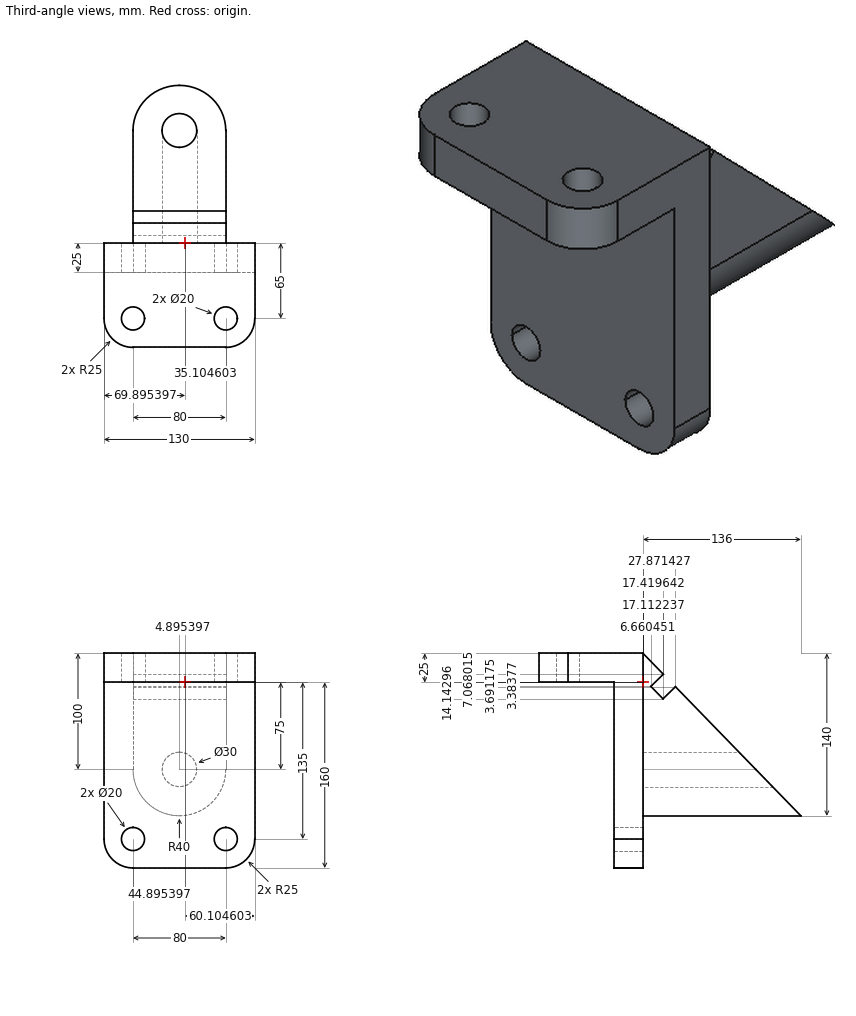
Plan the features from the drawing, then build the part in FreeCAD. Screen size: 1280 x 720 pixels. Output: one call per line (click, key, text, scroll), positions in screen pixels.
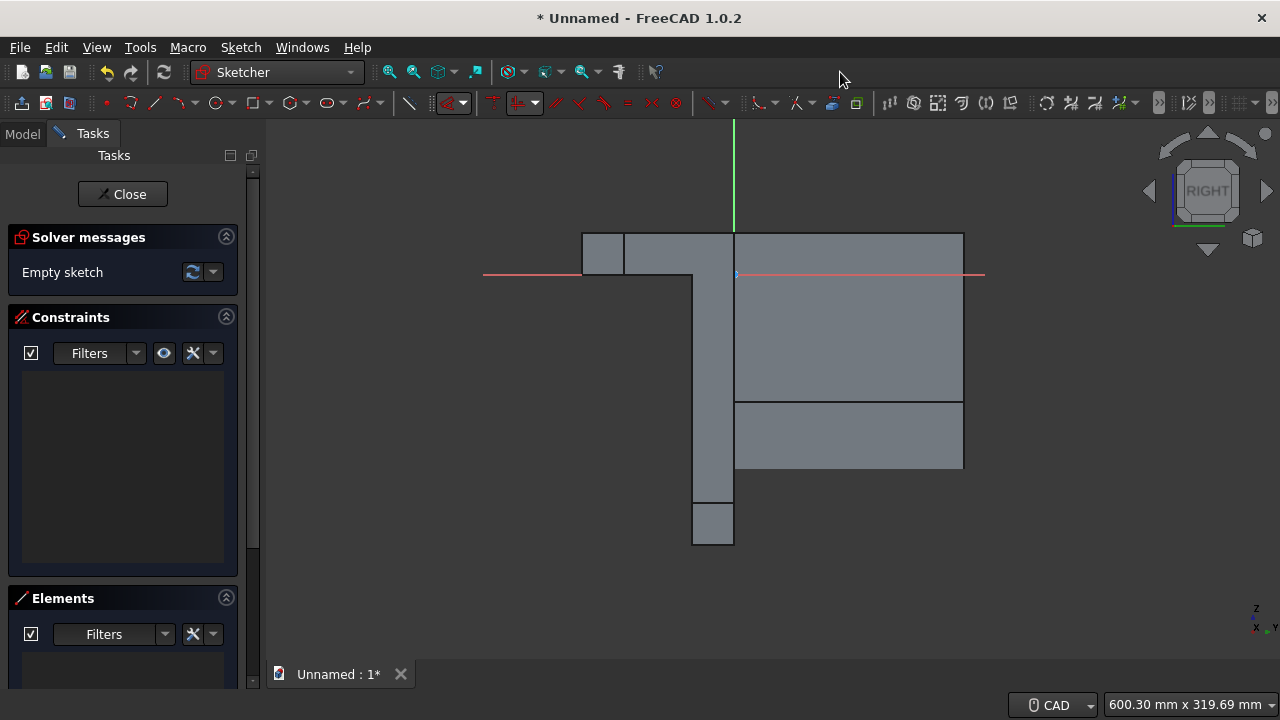
click(70, 104)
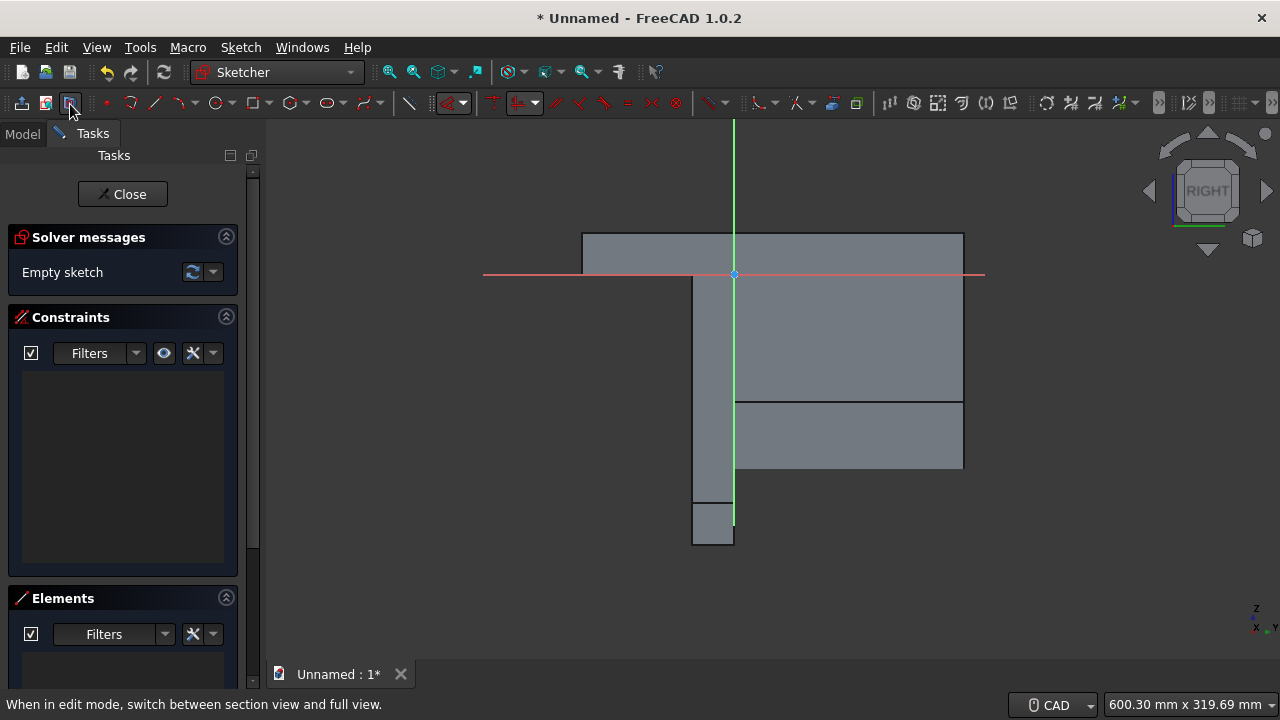
scroll(1115, 274, up, 2)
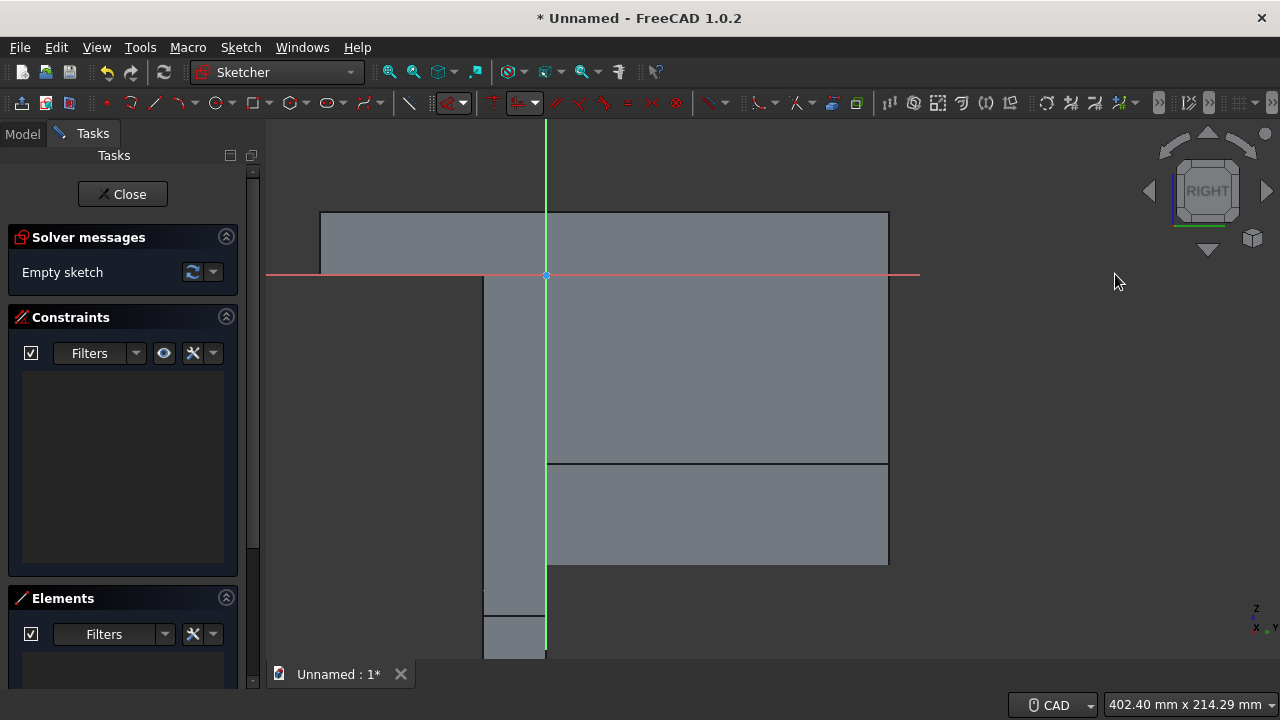
click(132, 104)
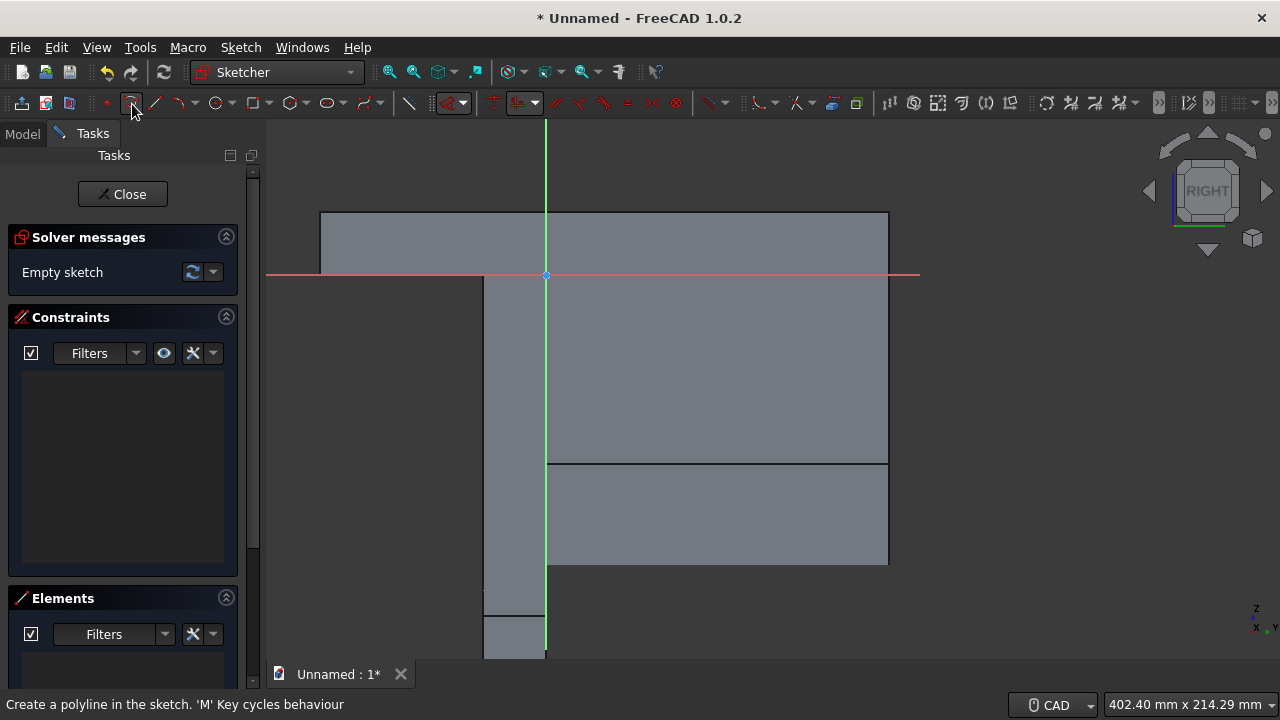
click(546, 212)
click(889, 565)
click(889, 212)
click(546, 213)
key(Escape)
key(Escape)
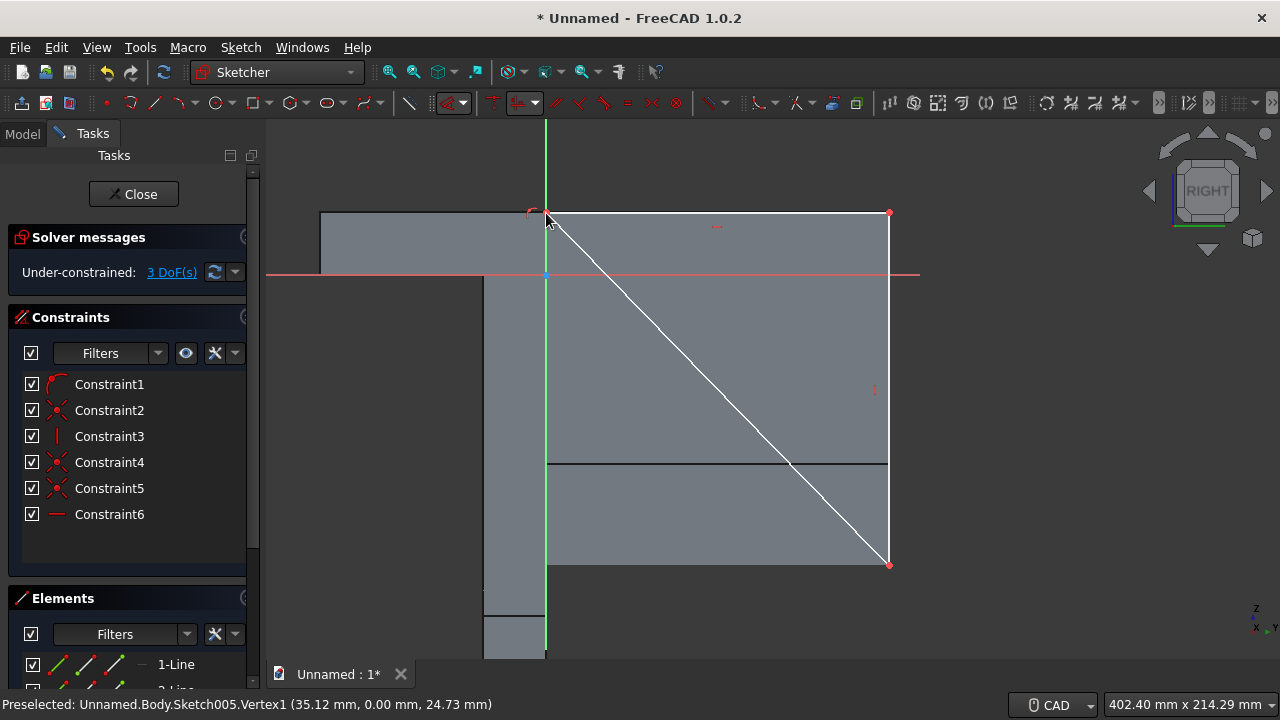
click(889, 460)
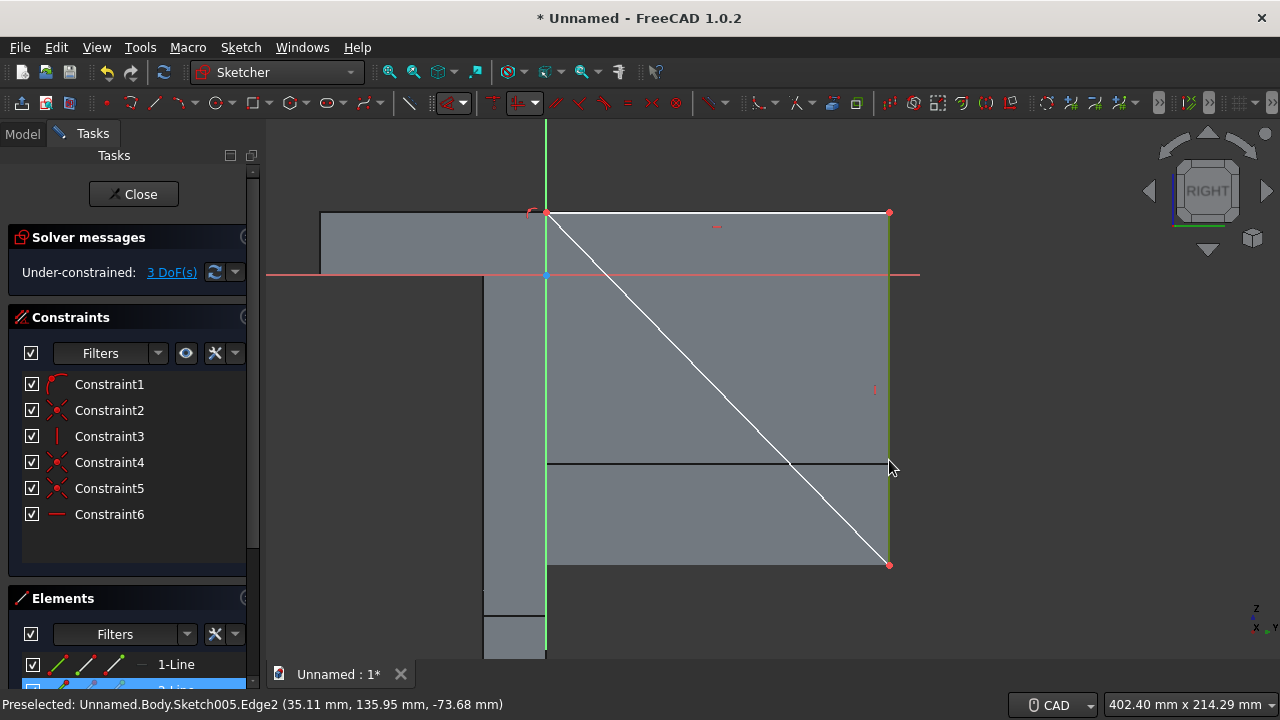
key(i)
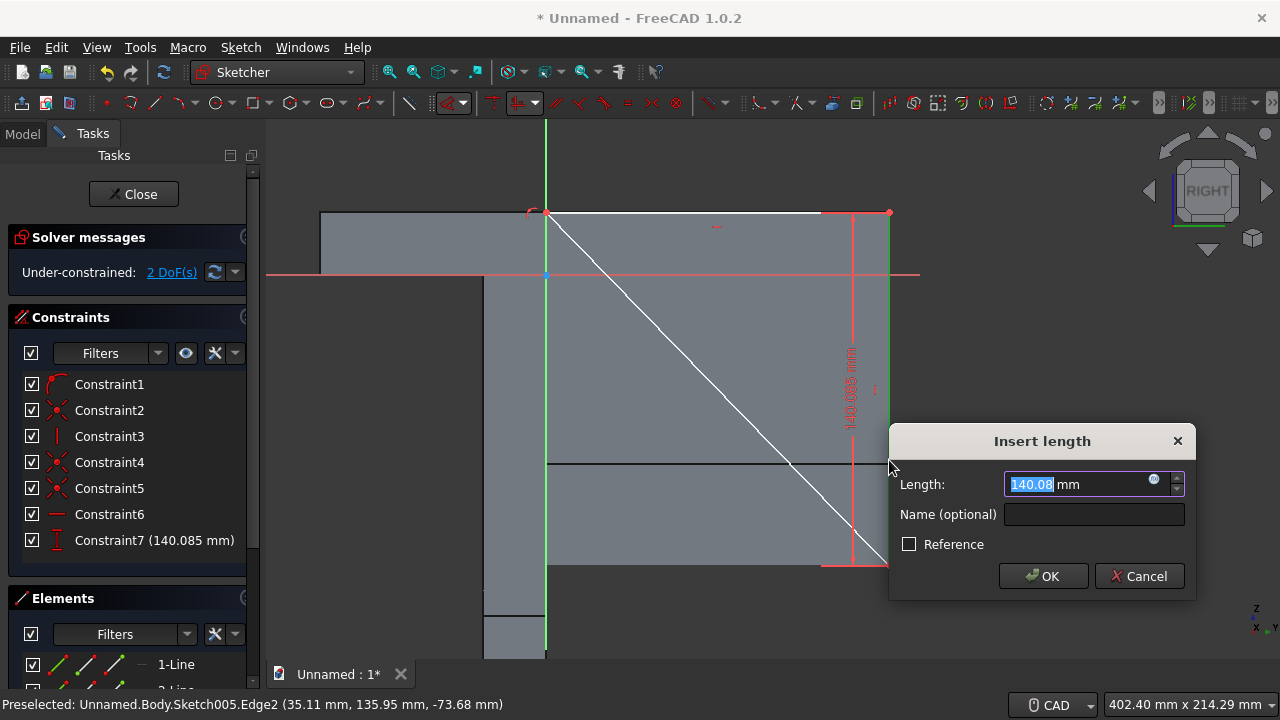
text(140)
key(Return)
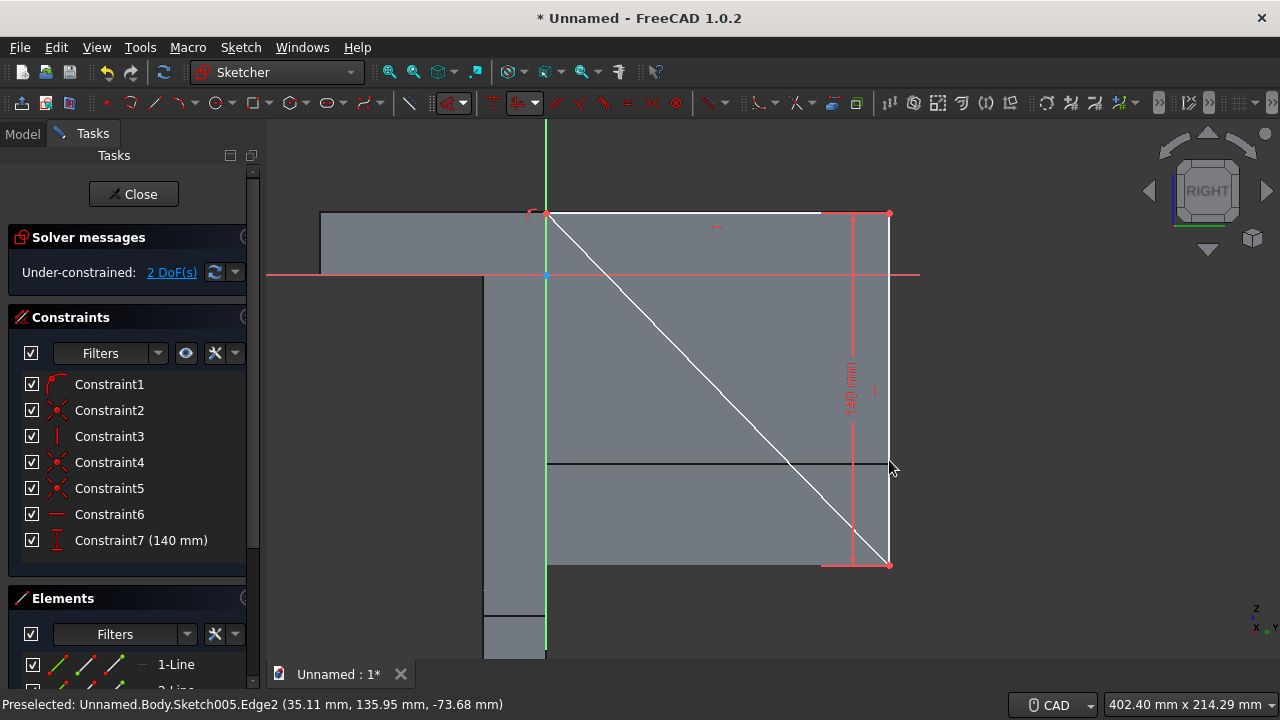
click(786, 213)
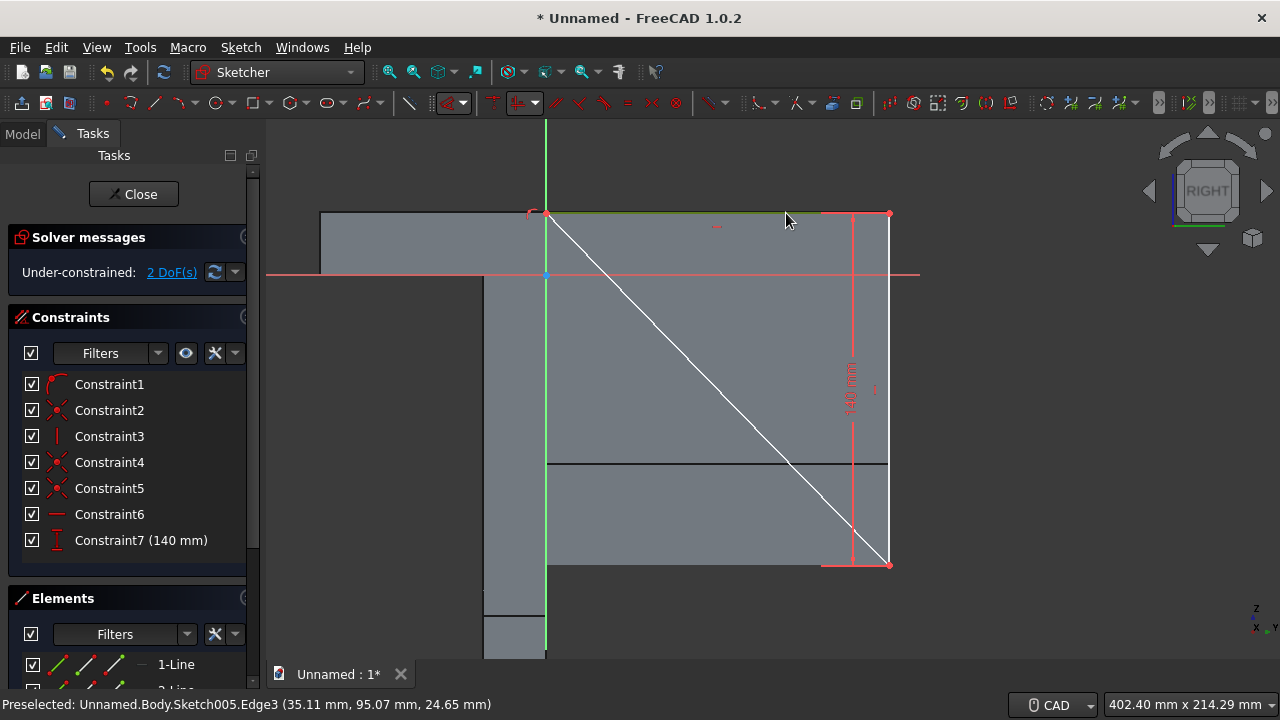
key(l)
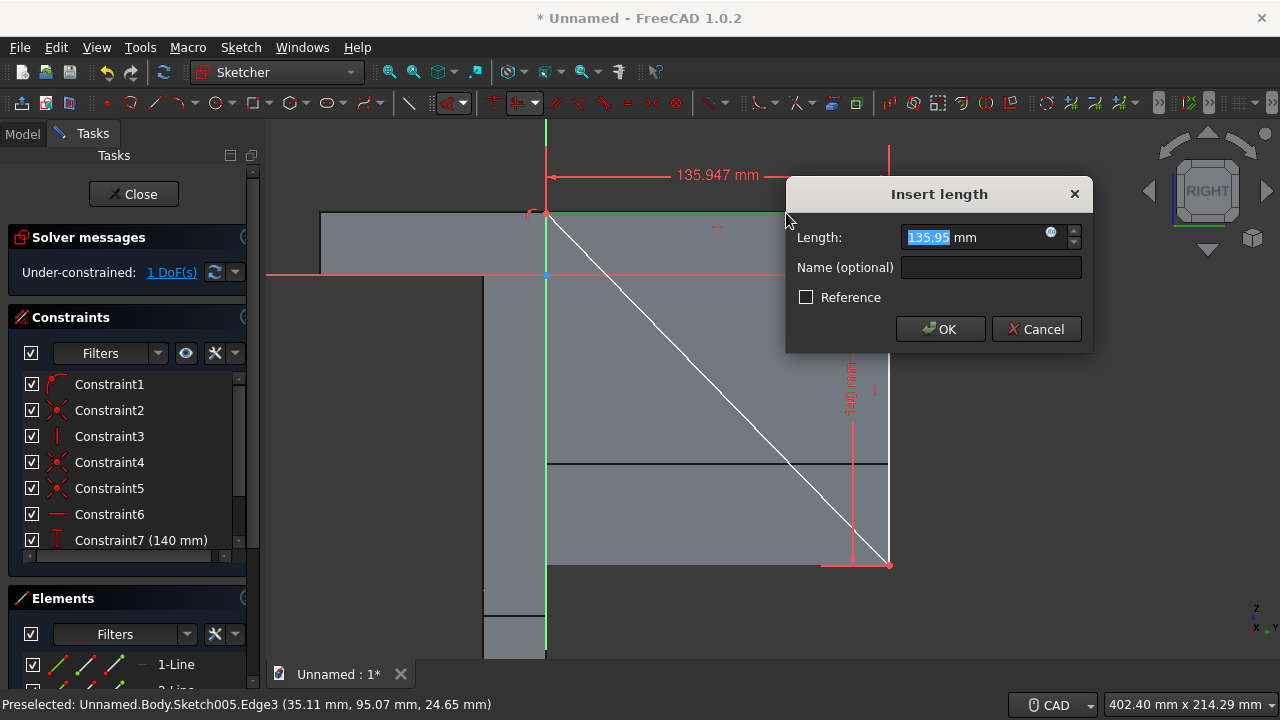
text(136)
key(Return)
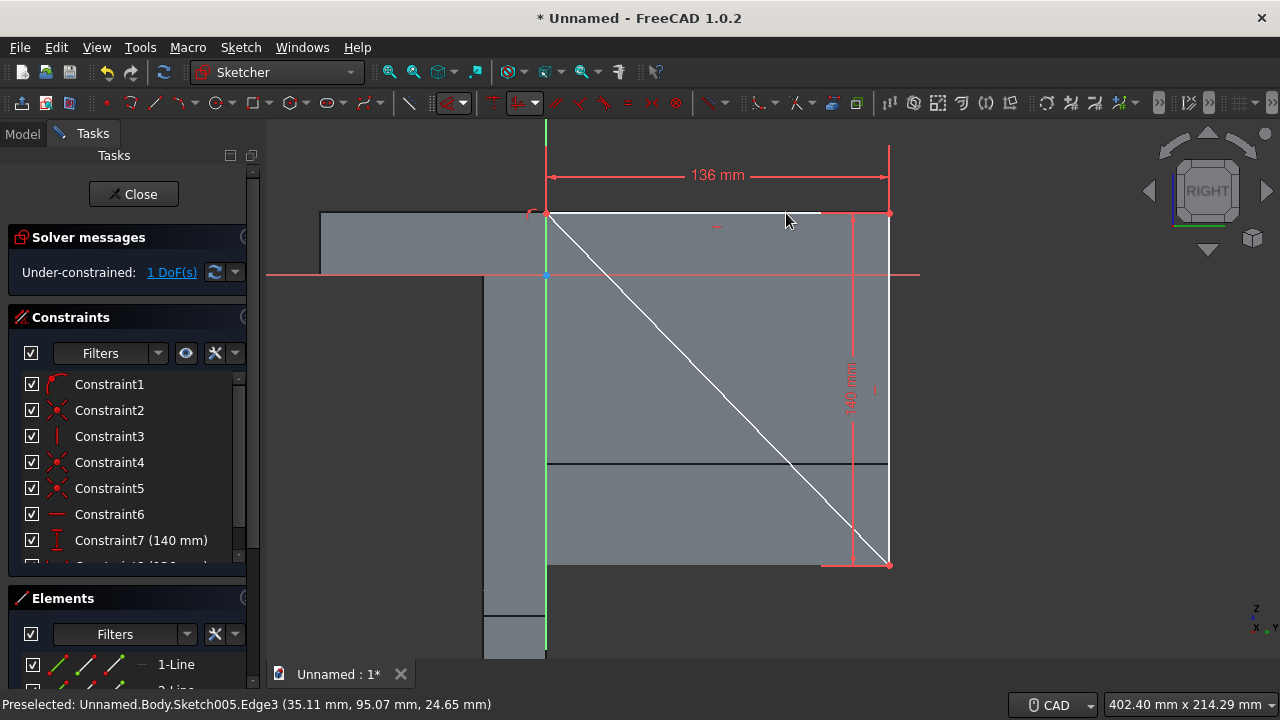
click(546, 213)